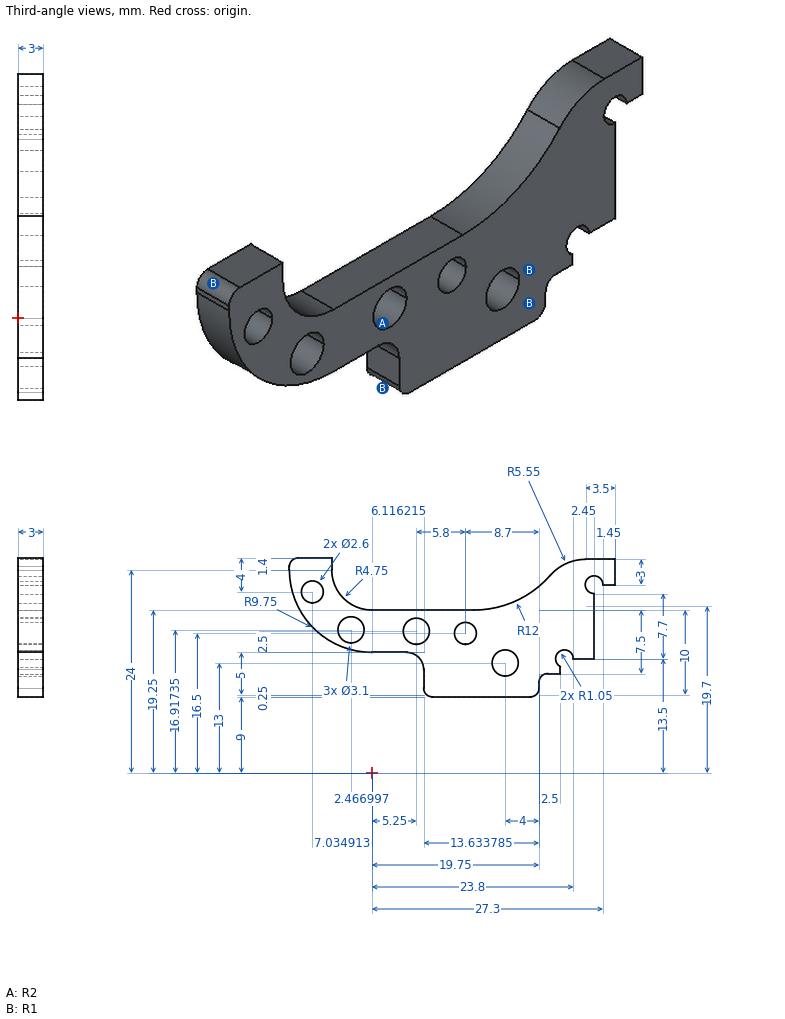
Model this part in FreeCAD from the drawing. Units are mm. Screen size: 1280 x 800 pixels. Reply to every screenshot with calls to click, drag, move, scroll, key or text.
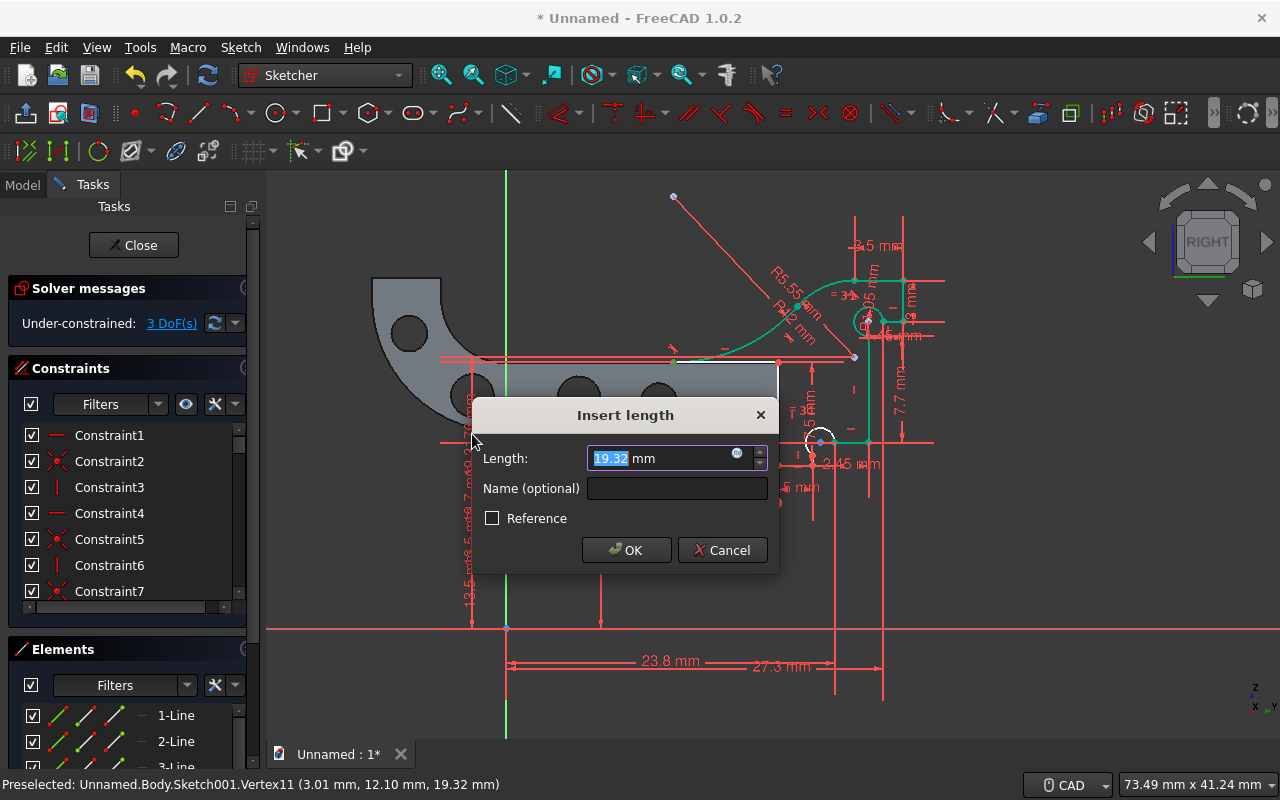
text(19.25)
key(Return)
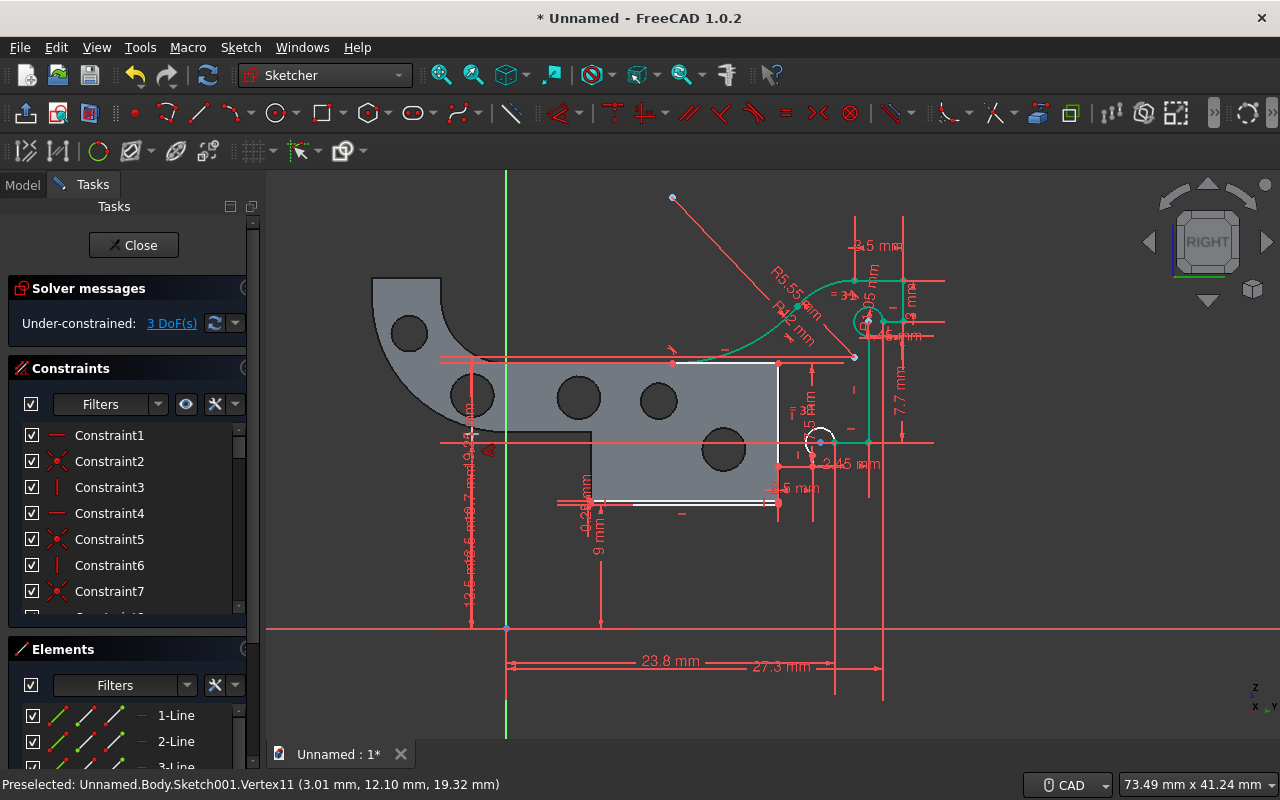
click(778, 363)
click(580, 663)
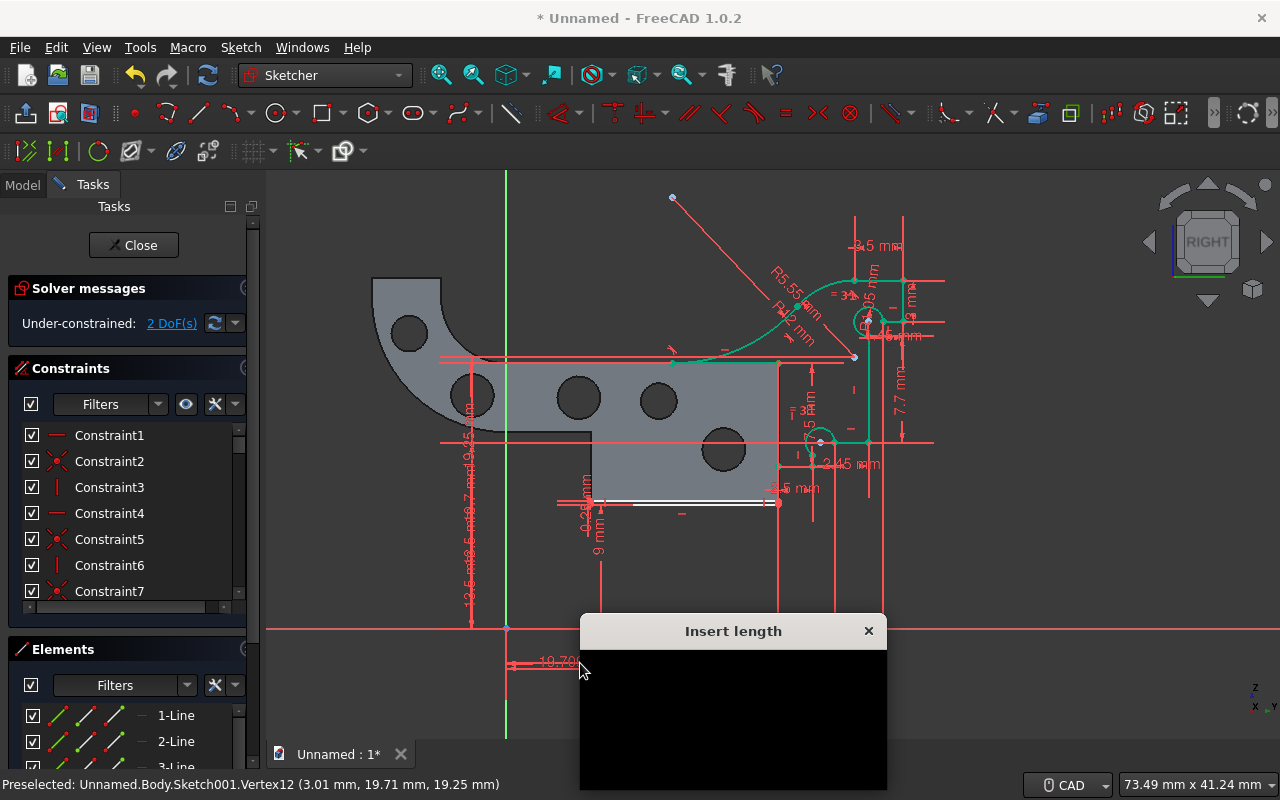
text(19.75)
key(Return)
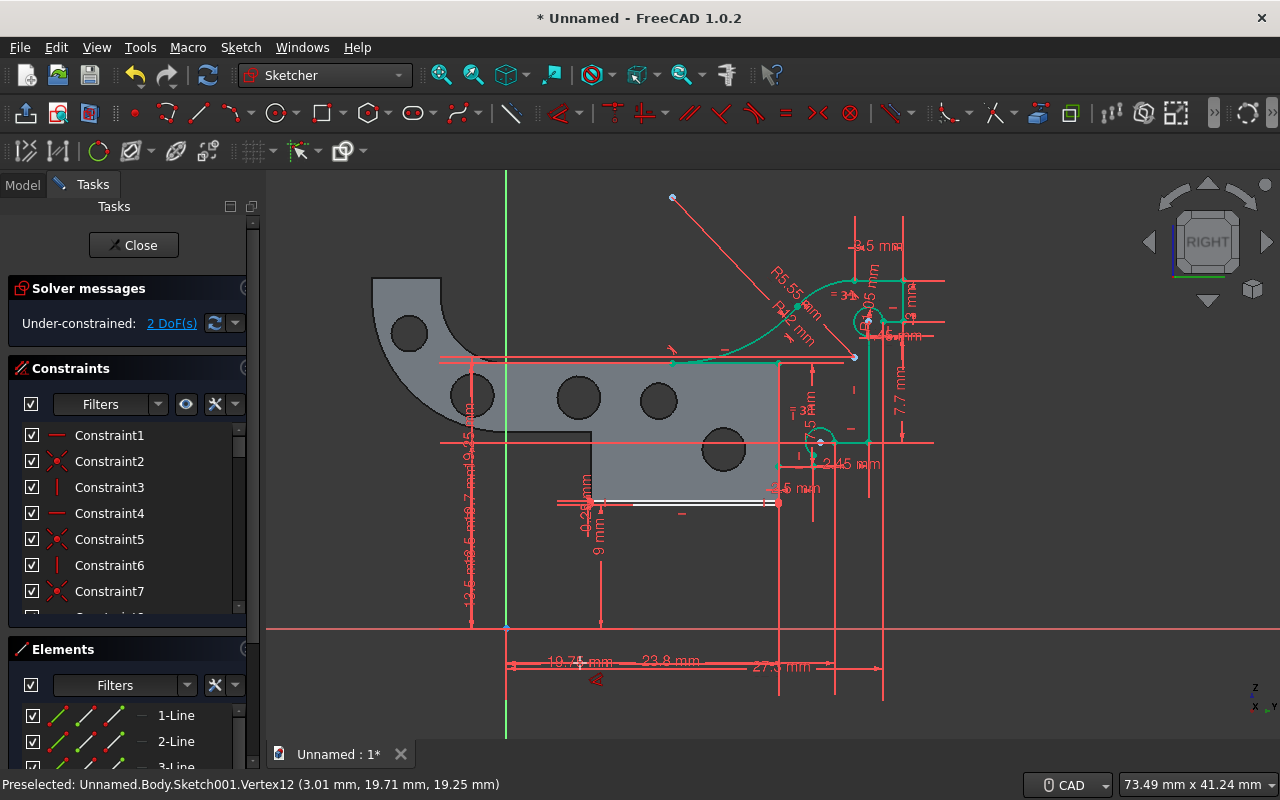
scroll(779, 505, up, 7)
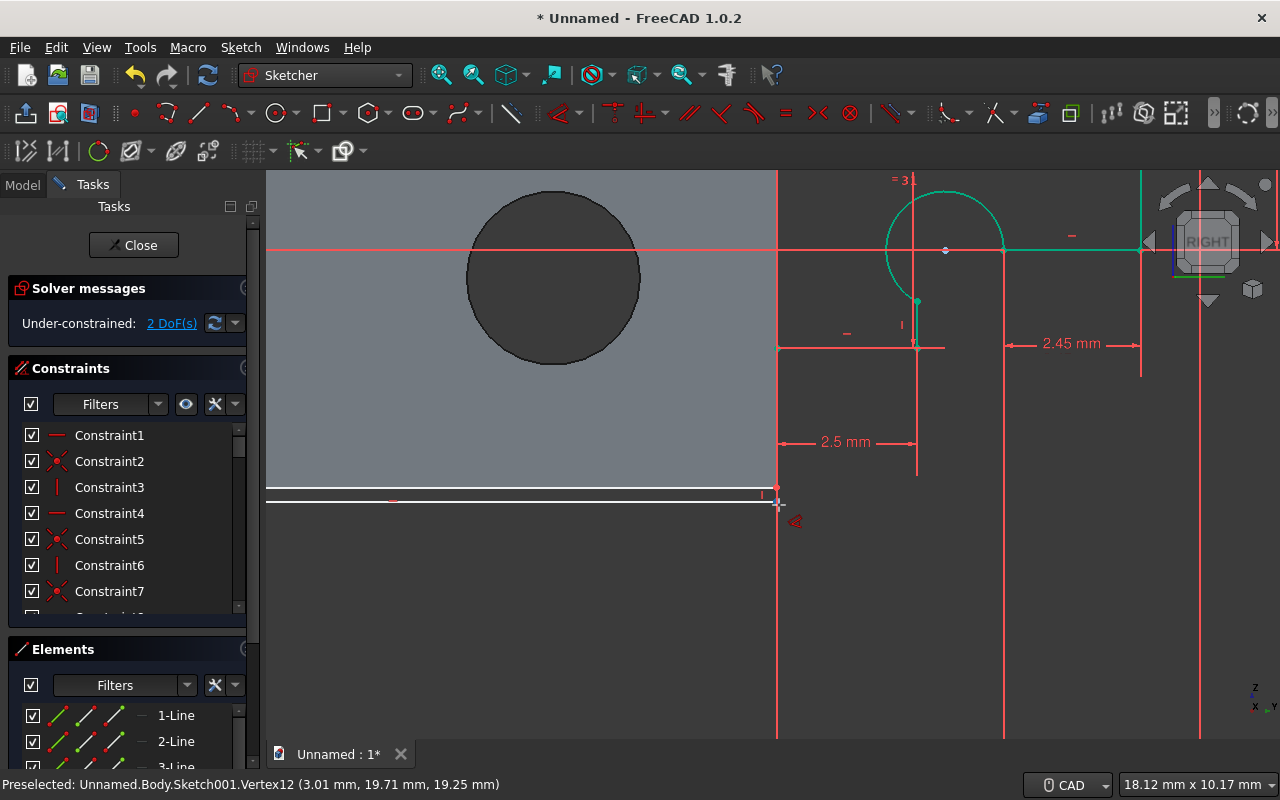
click(777, 502)
click(535, 468)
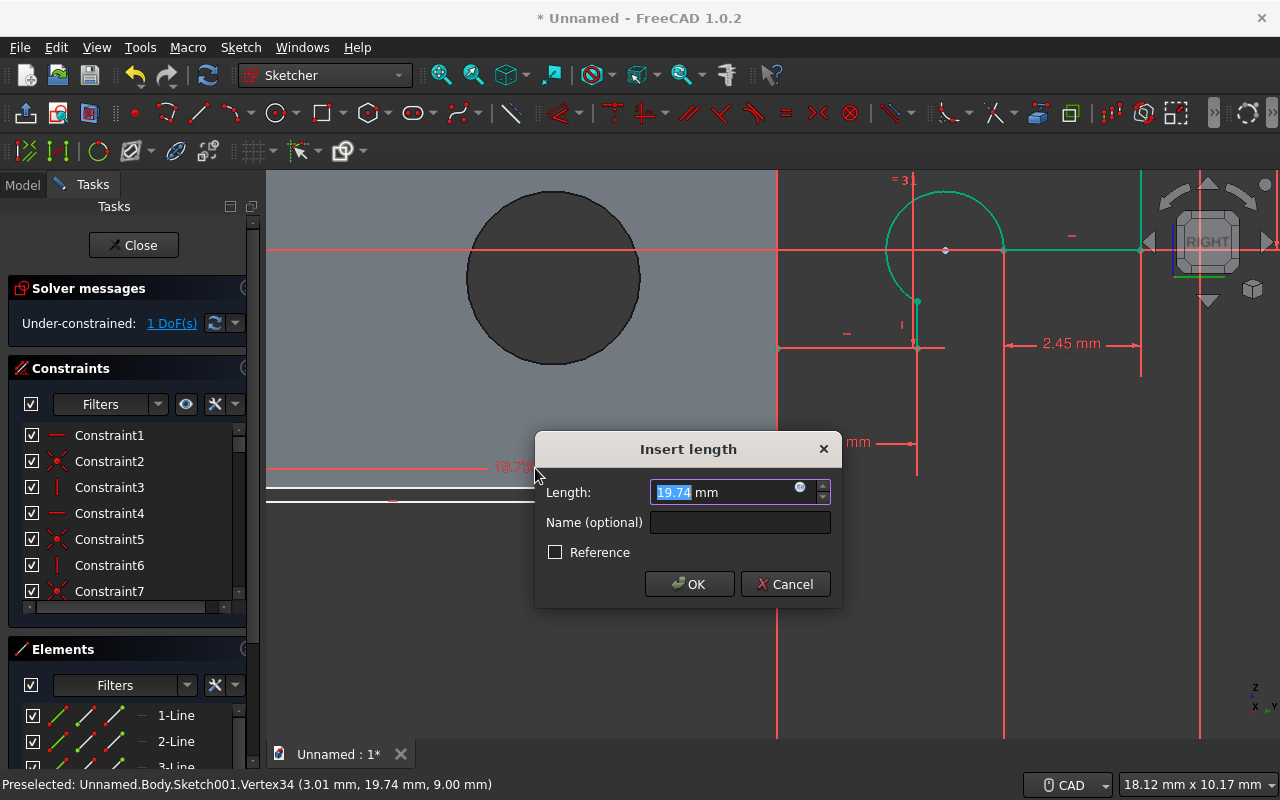
text(19.75)
key(Return)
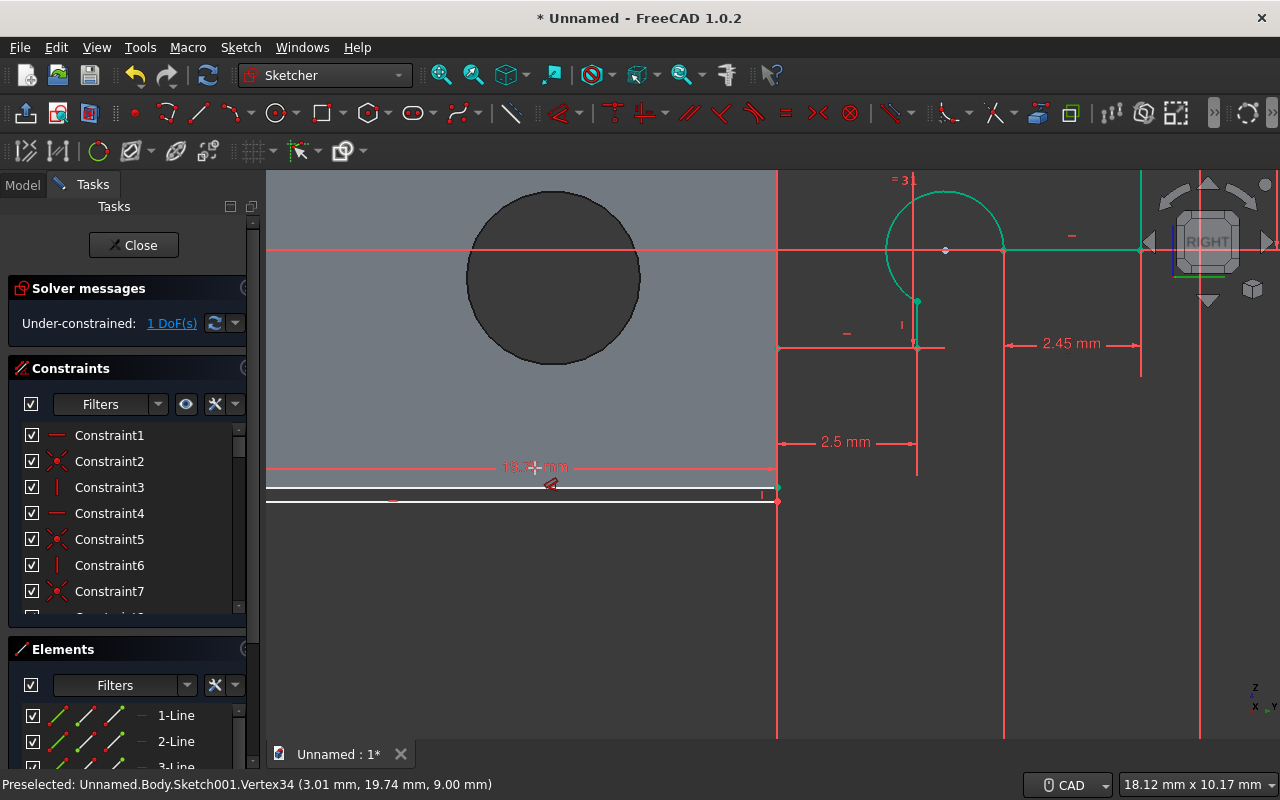
click(548, 502)
click(536, 536)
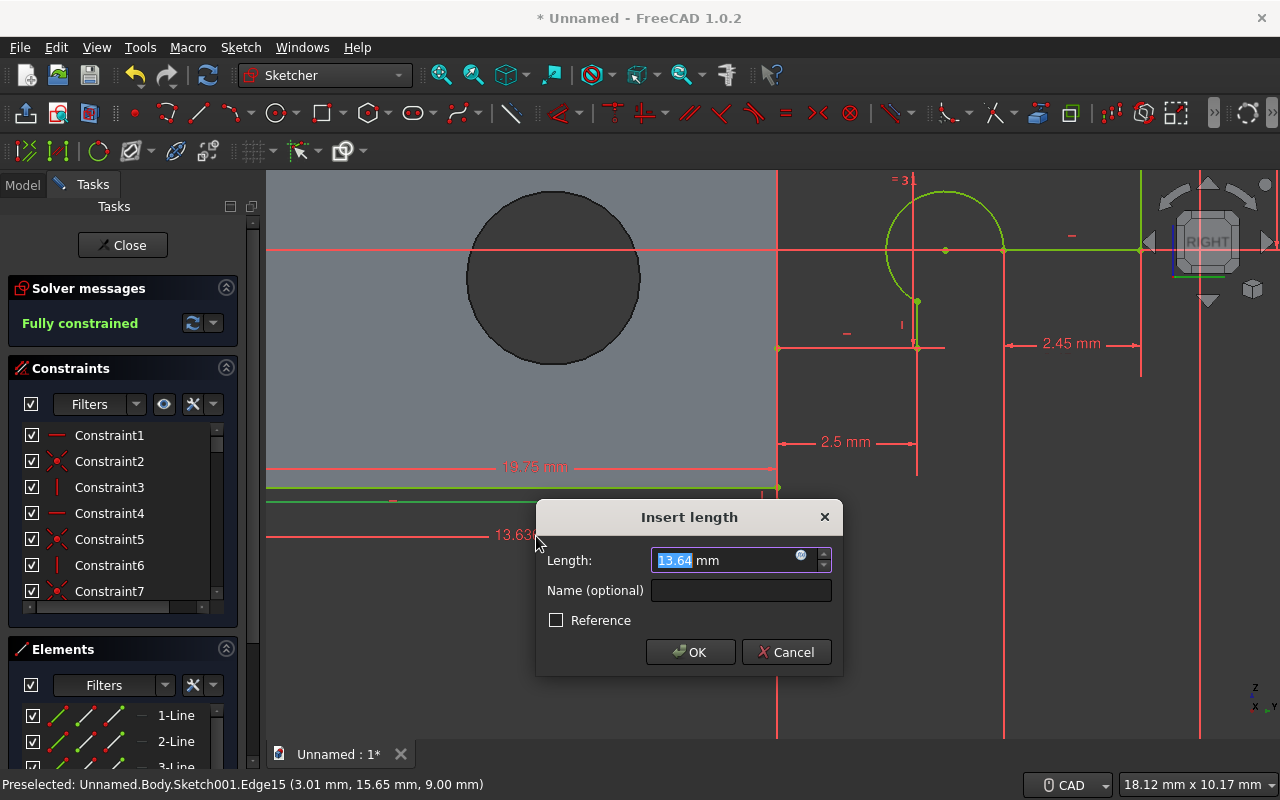
text(13.633785)
key(Return)
key(Escape)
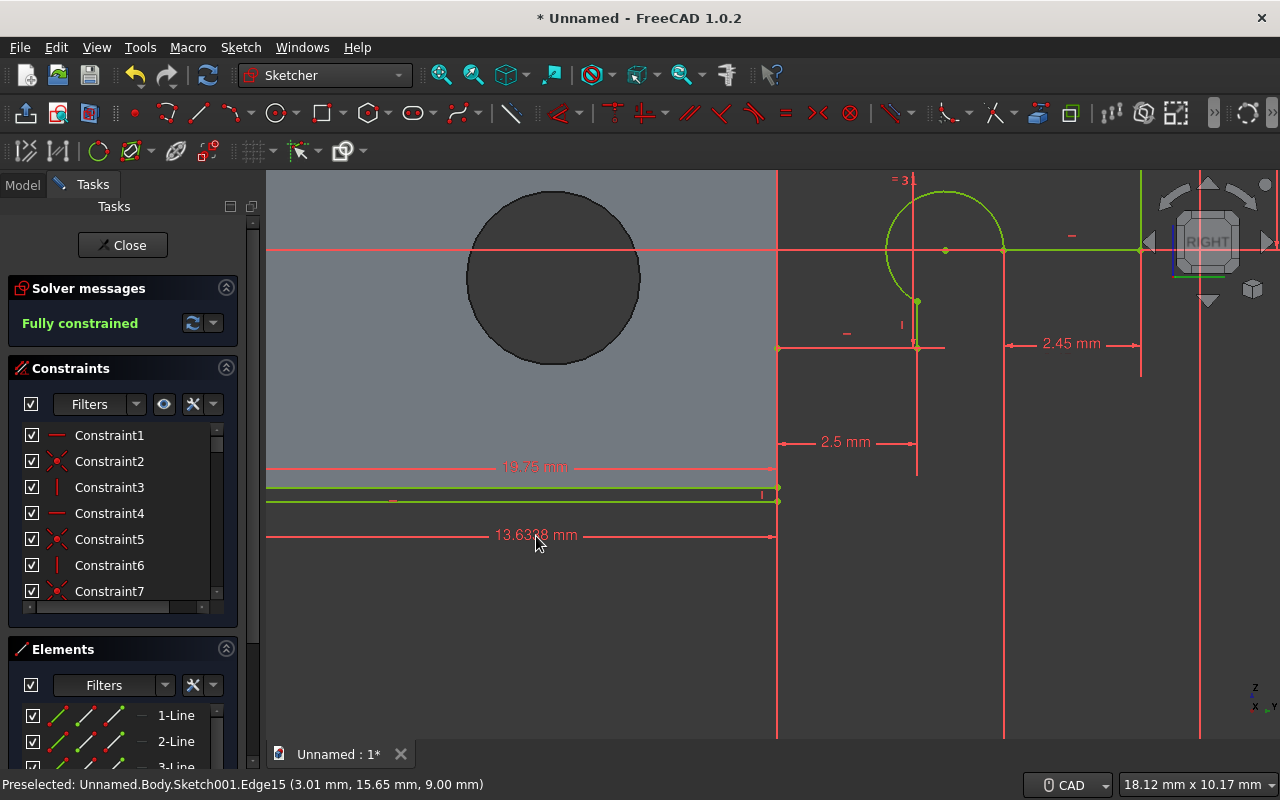
click(123, 245)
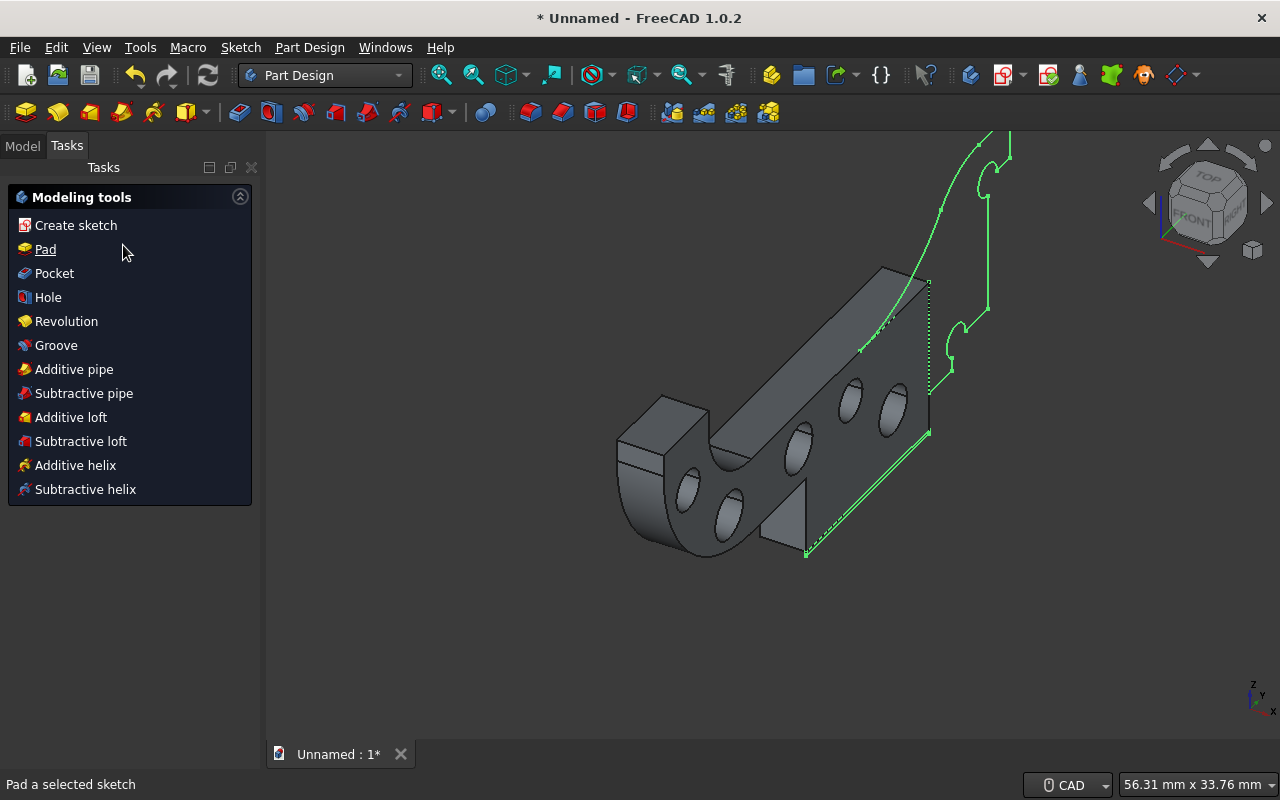
click(26, 112)